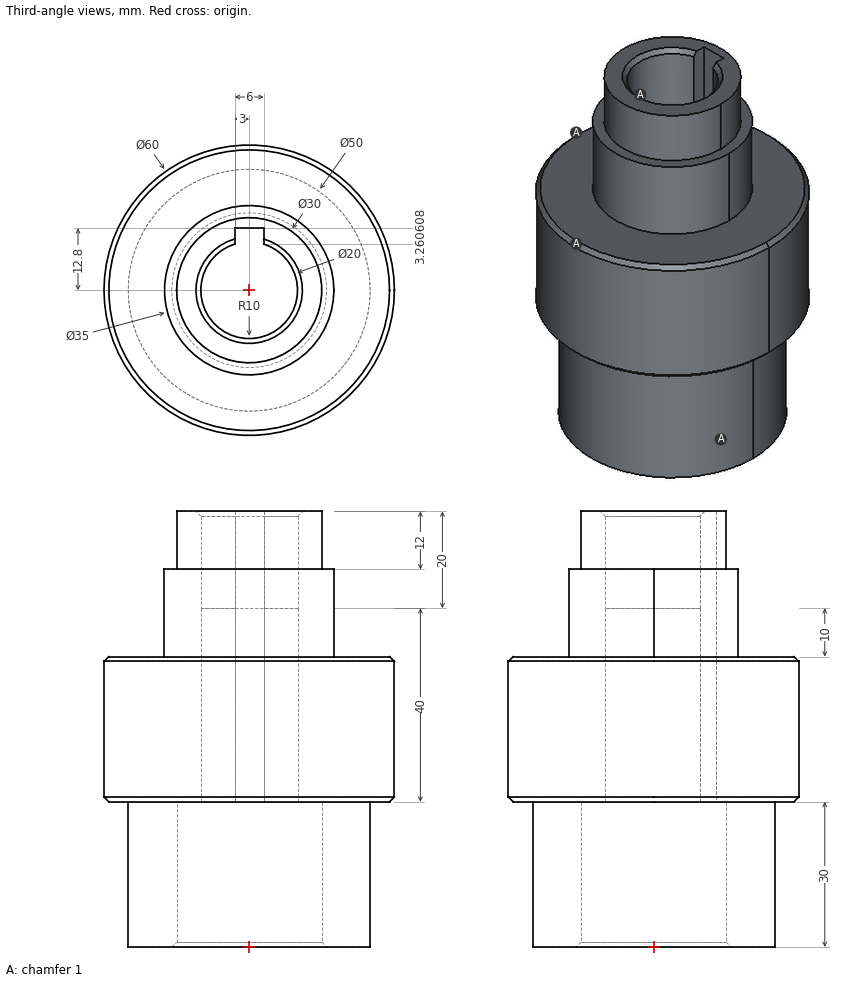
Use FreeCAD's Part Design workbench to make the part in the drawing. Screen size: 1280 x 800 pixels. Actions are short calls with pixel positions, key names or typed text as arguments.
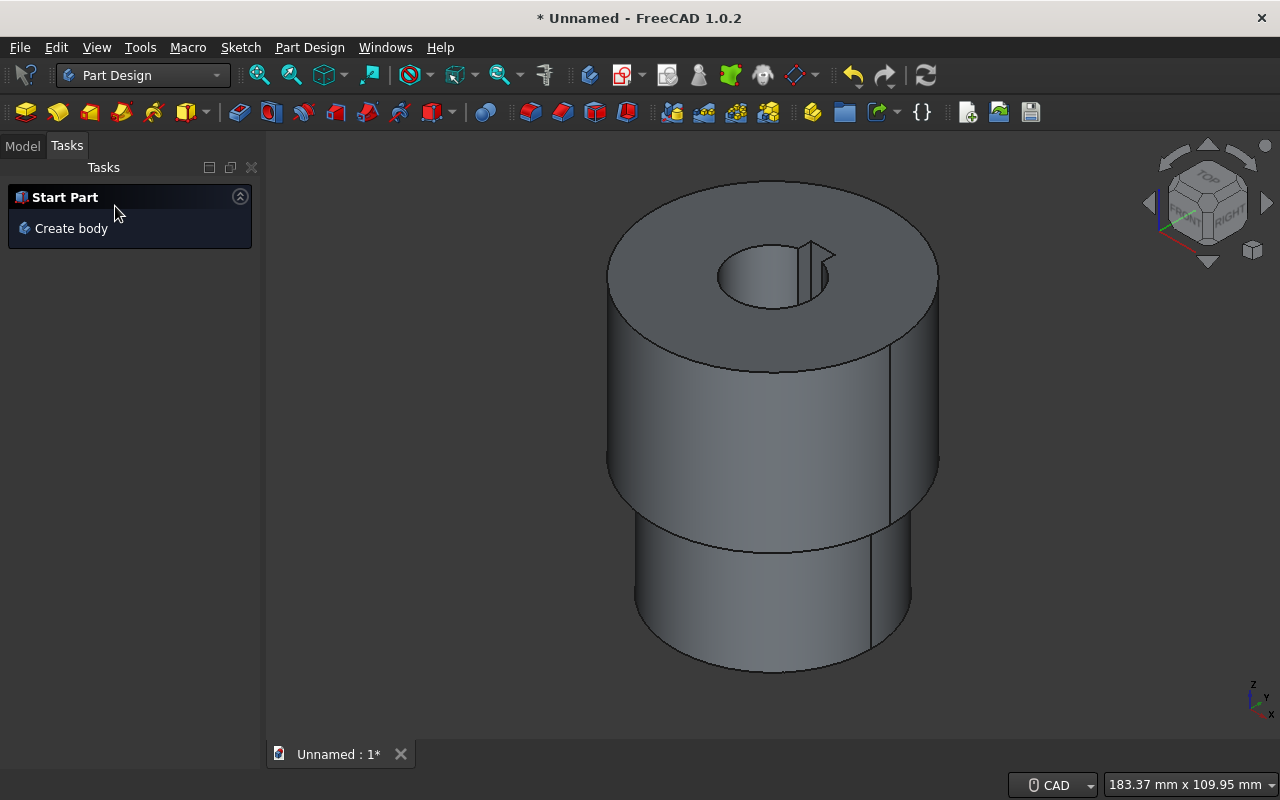
key(5)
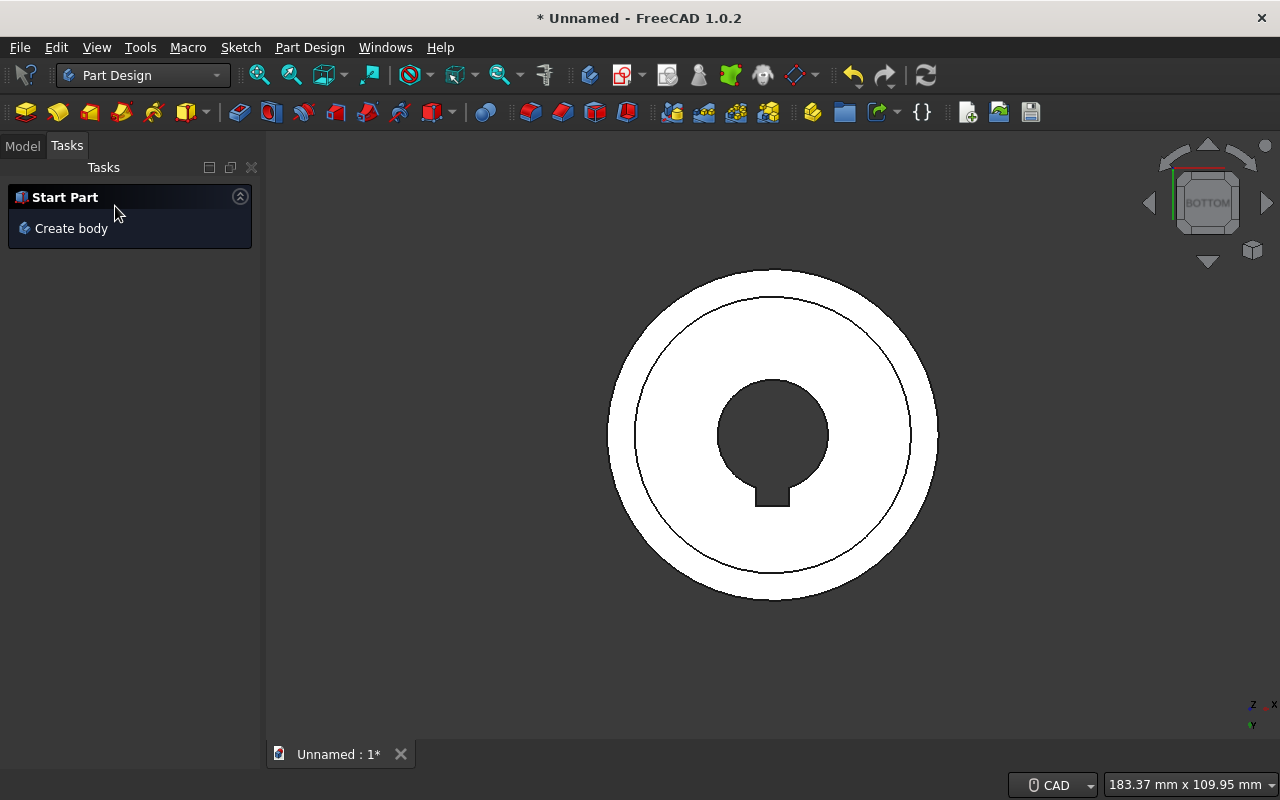
click(694, 473)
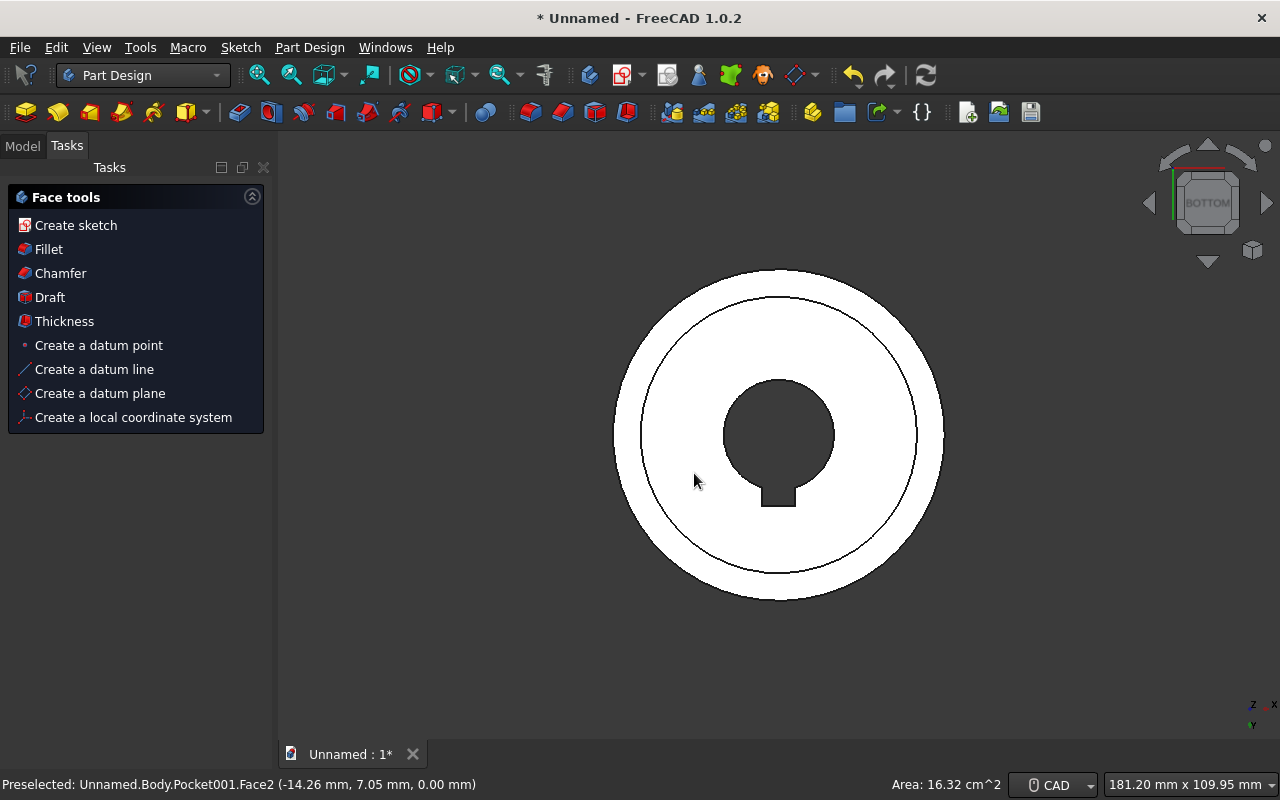
click(622, 76)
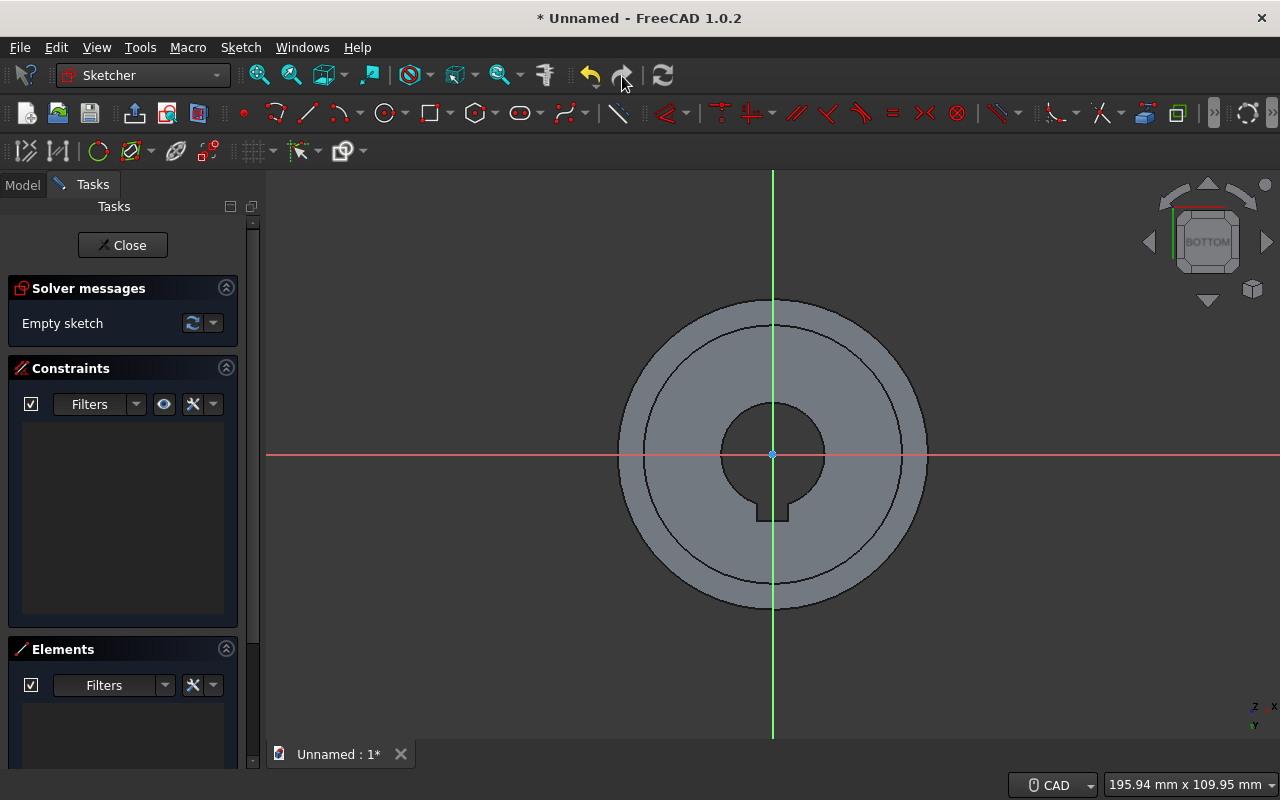
scroll(829, 455, up, 4)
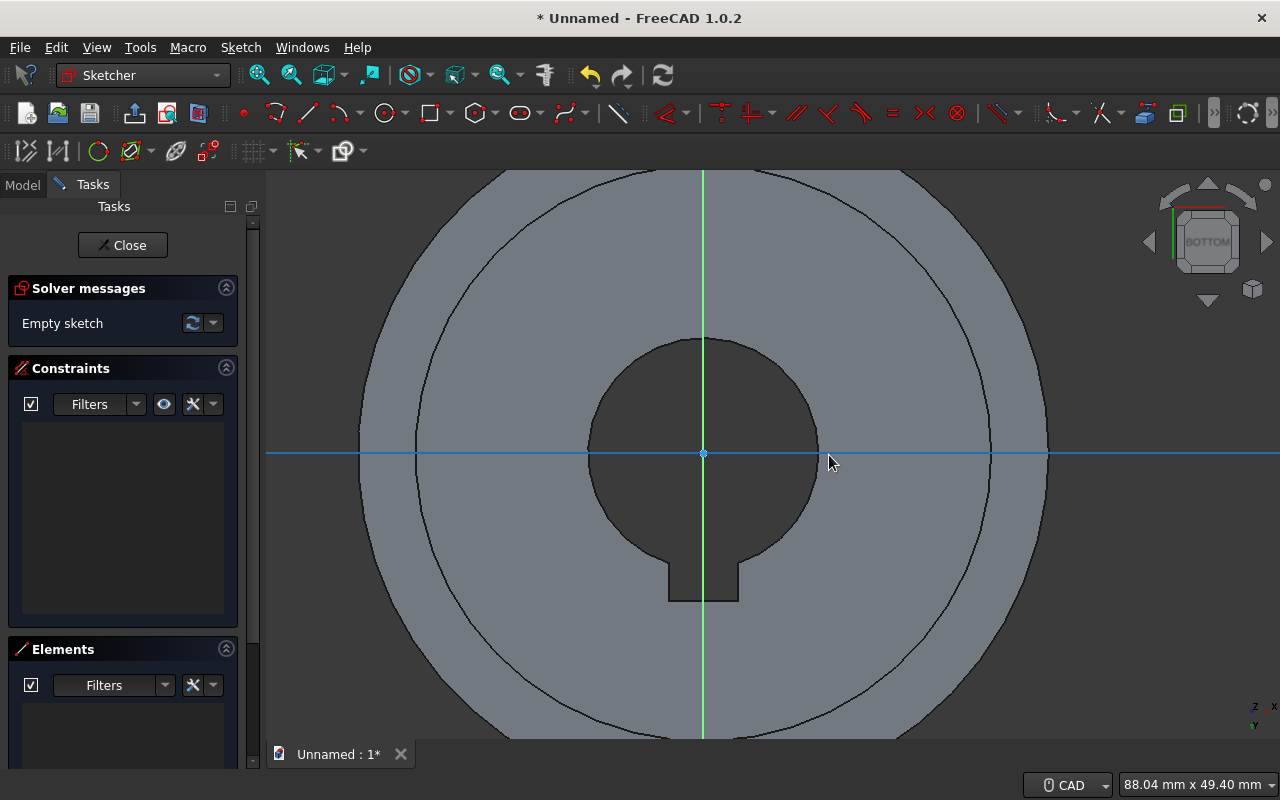
click(386, 114)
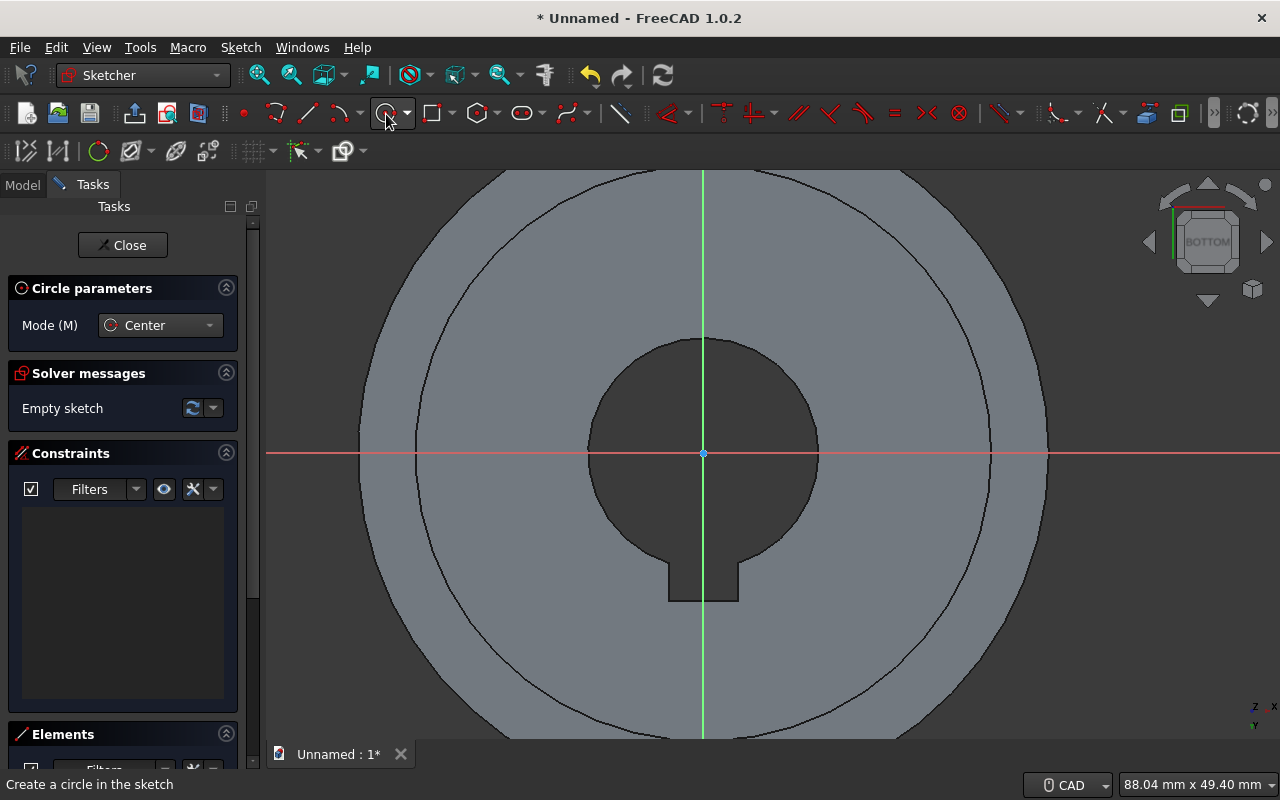
click(703, 453)
move(825, 331)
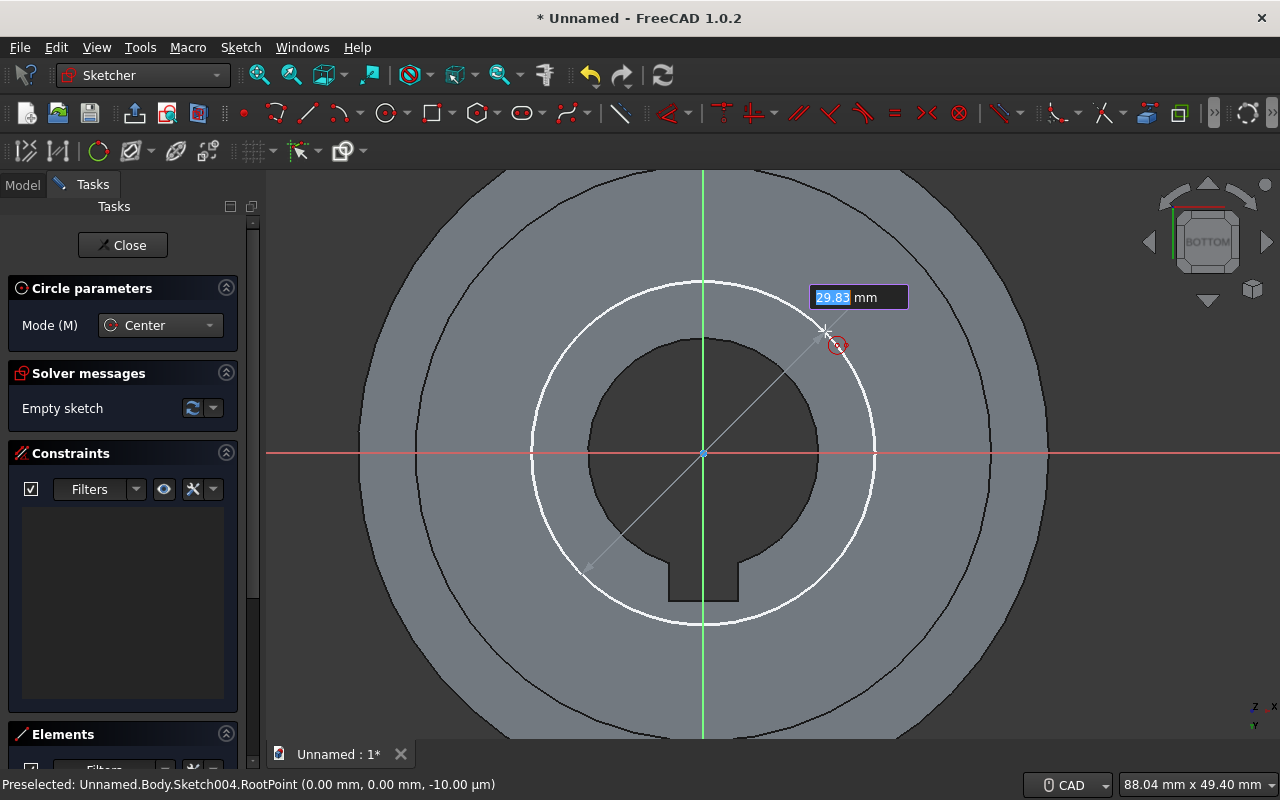
text(30)
key(Return)
key(Escape)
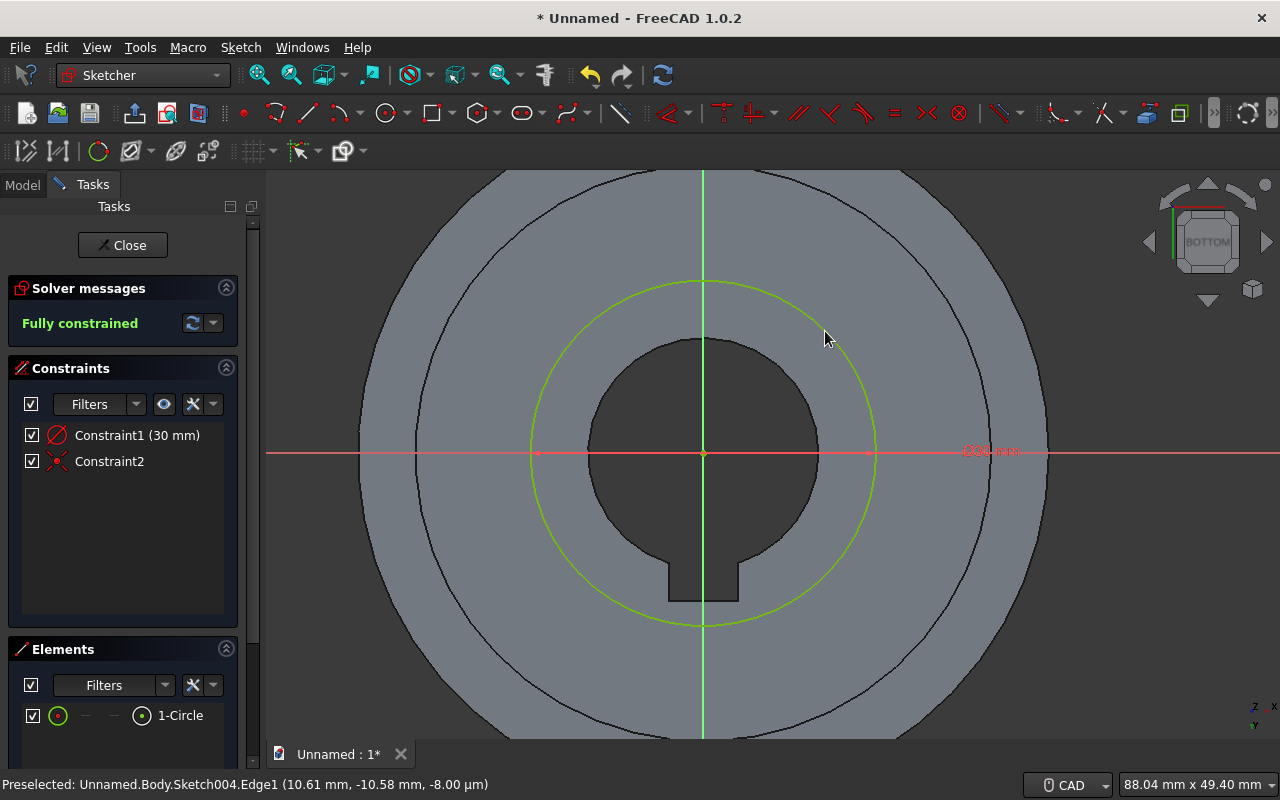
click(123, 245)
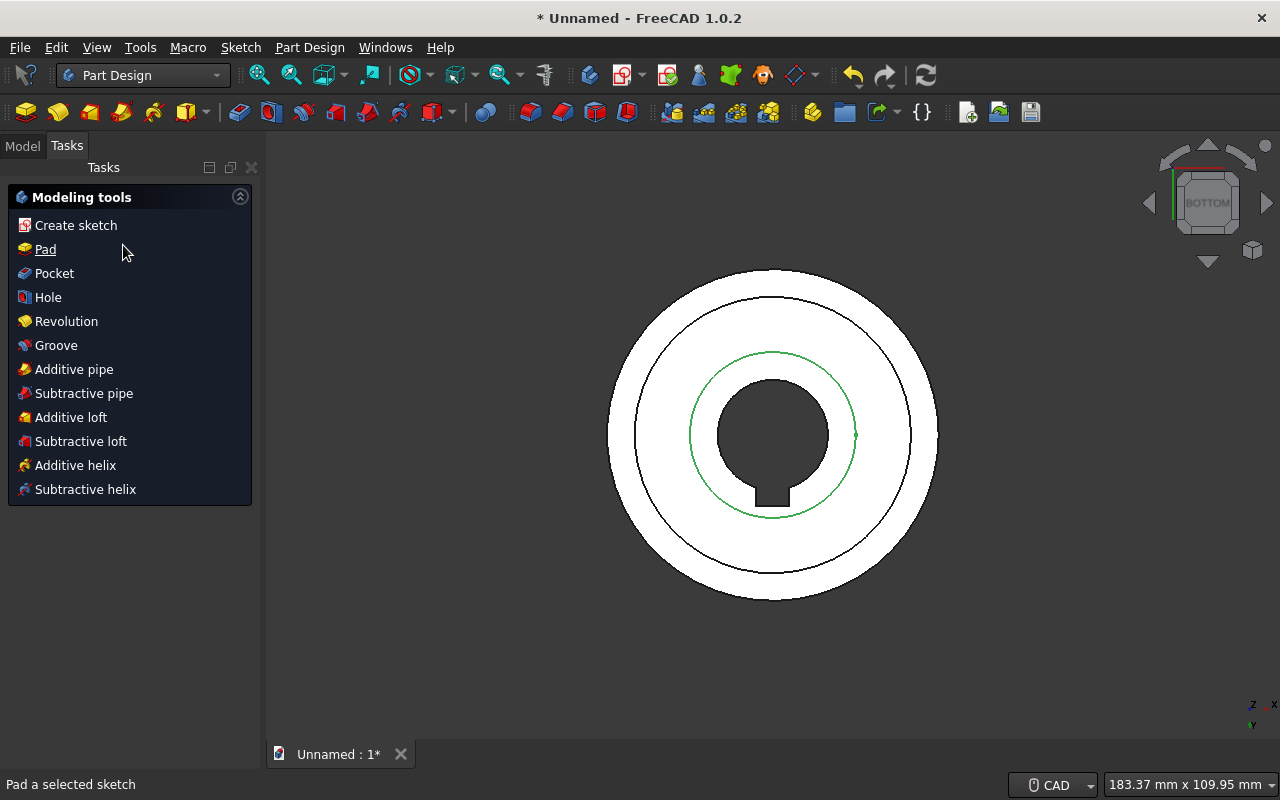
click(240, 112)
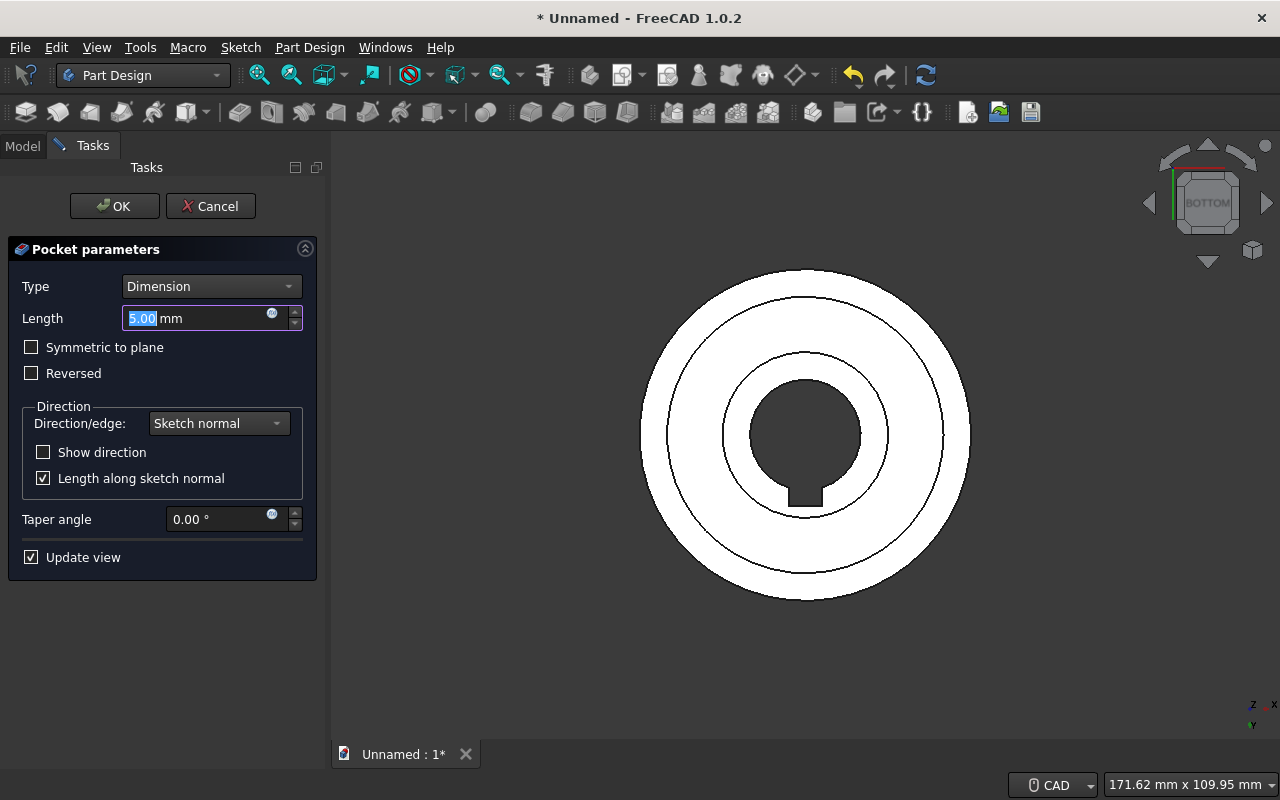
text(30)
key(Tab)